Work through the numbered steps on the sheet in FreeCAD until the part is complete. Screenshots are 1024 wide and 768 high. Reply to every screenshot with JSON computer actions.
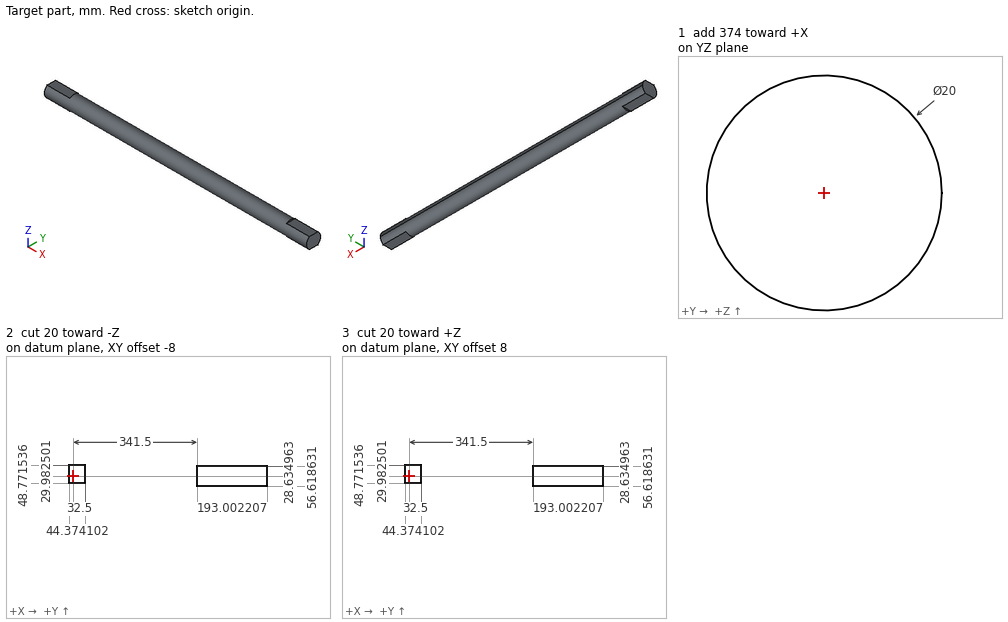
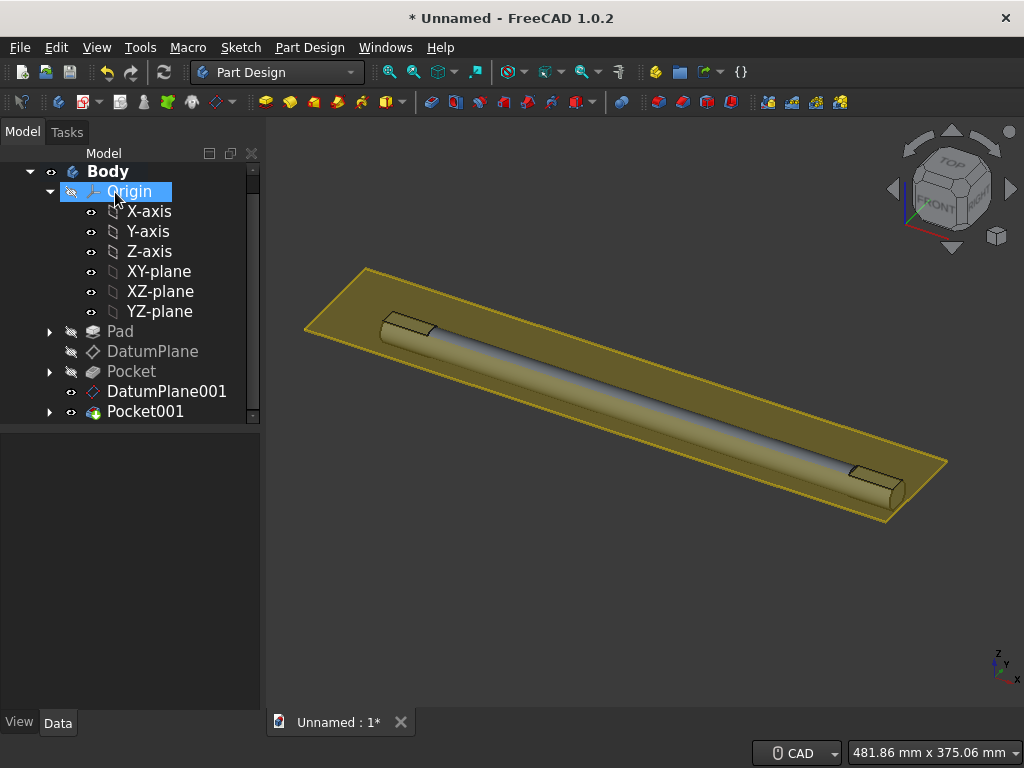
{"action": "left_click", "coordinate": [116, 392]}
{"action": "key", "text": "space"}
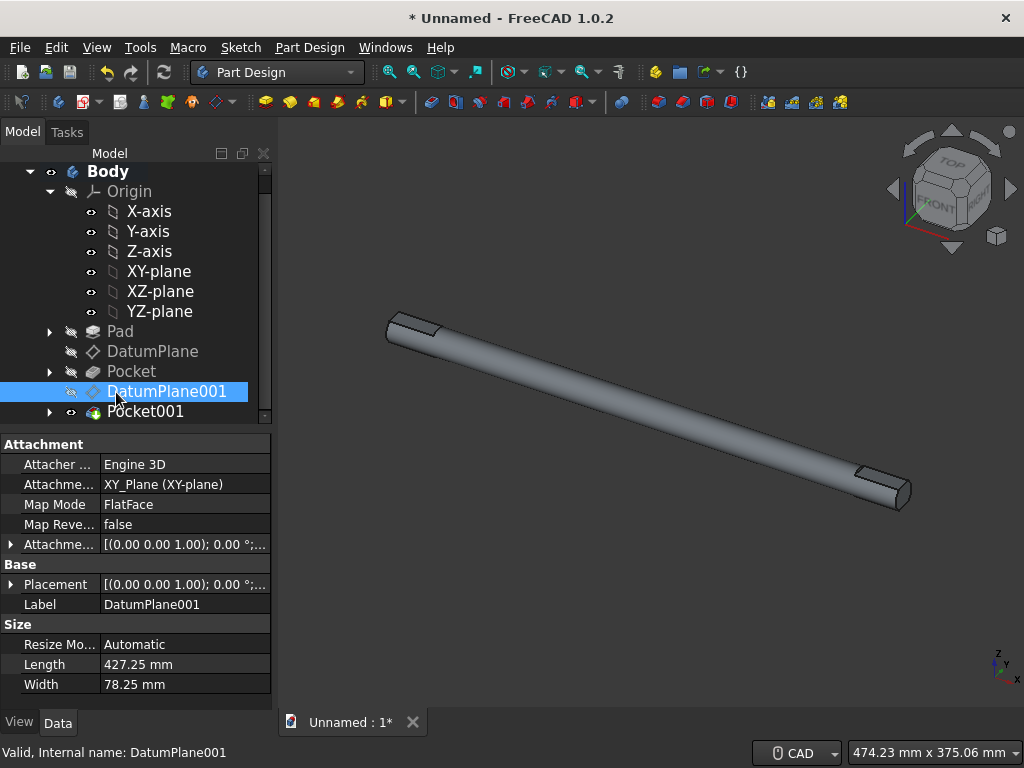
{"action": "key", "text": "0"}